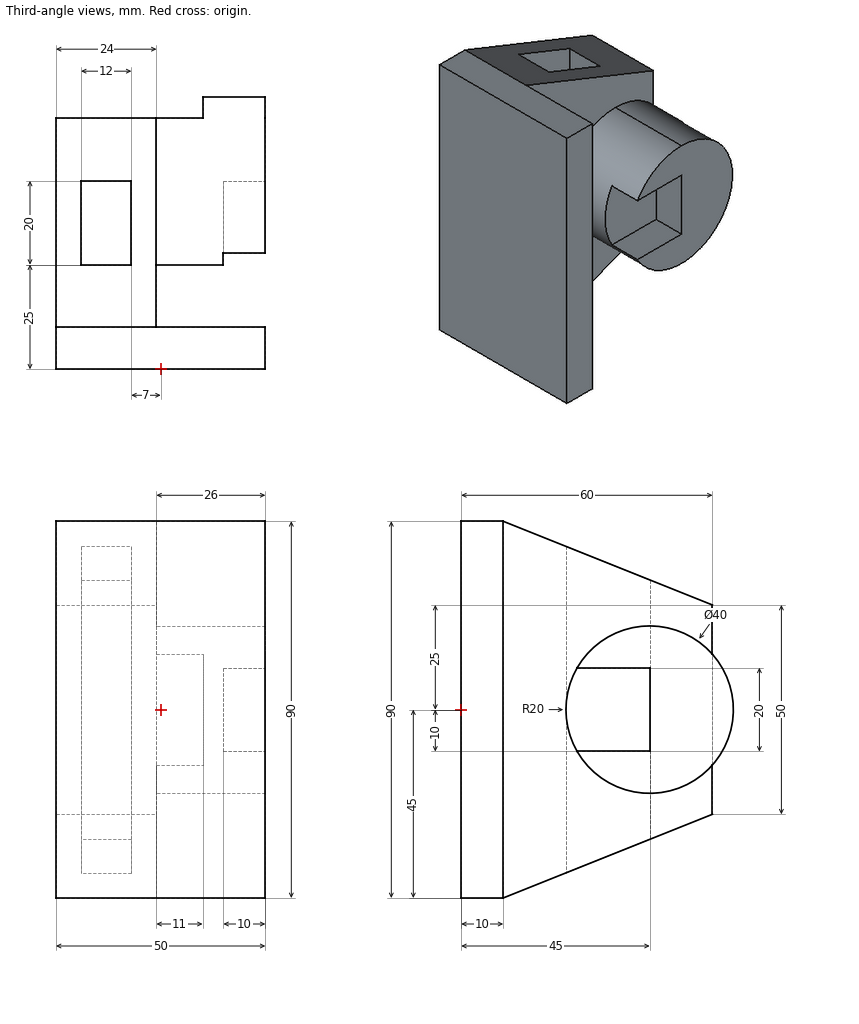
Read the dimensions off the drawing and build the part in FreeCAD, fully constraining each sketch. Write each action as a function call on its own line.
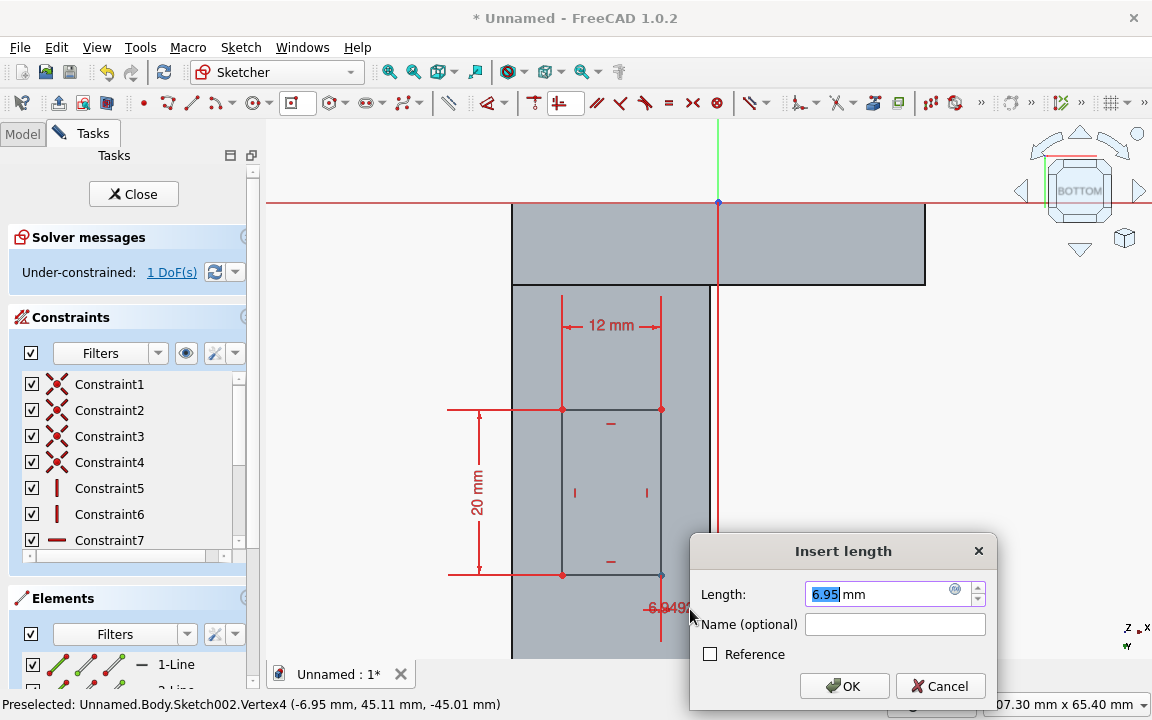
text(7)
key(Return)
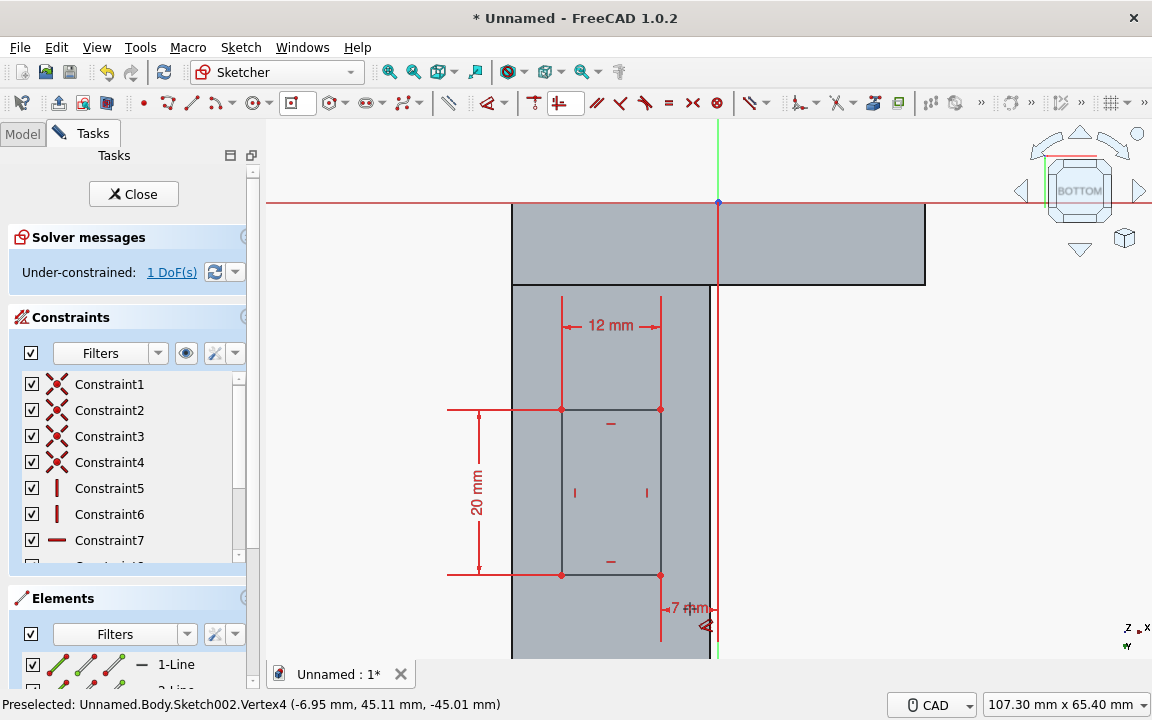
click(562, 410)
click(752, 306)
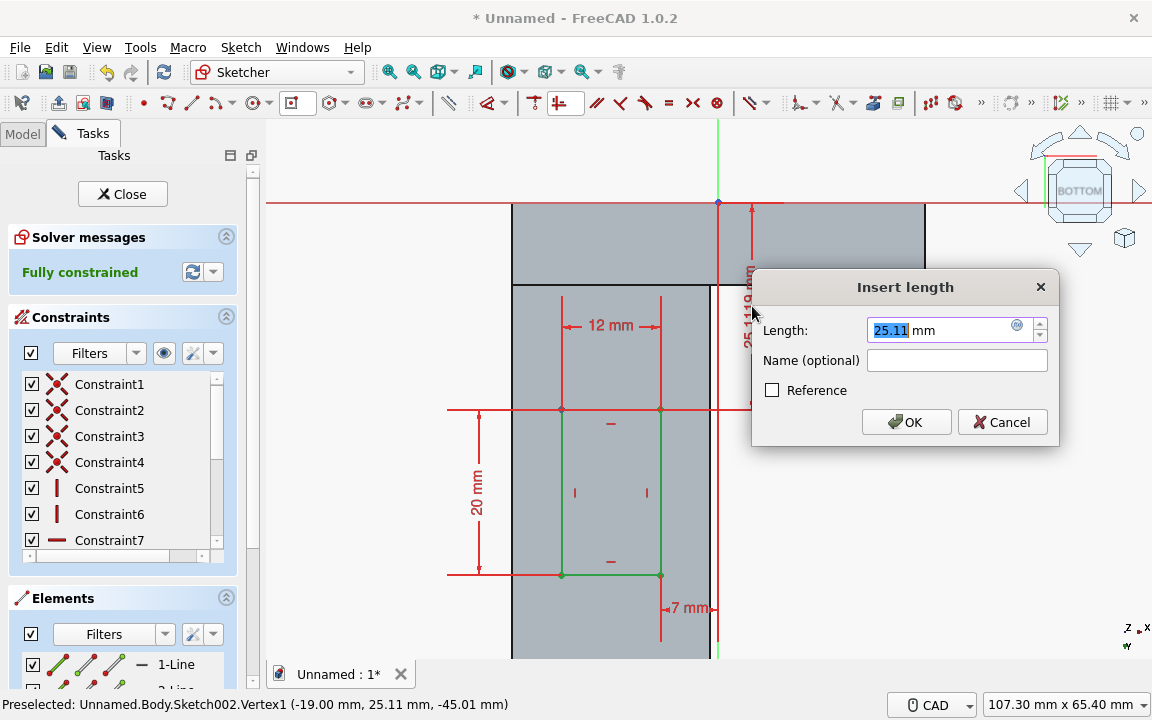
text(25)
key(Return)
key(Escape)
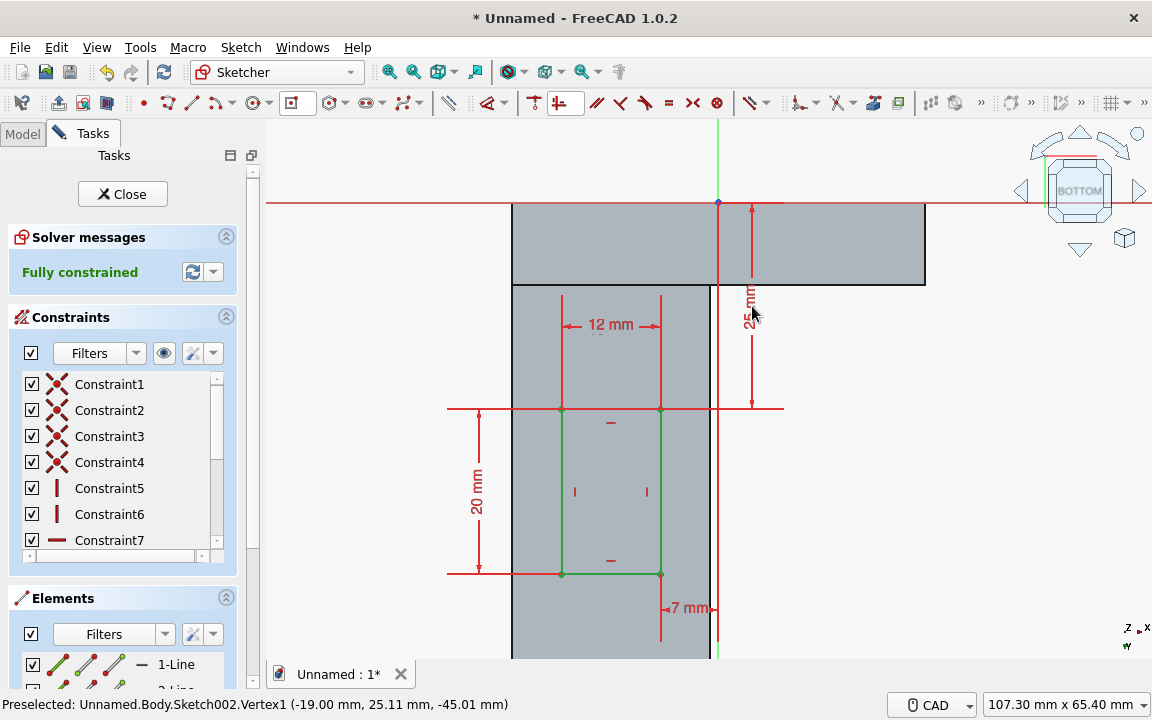
click(123, 194)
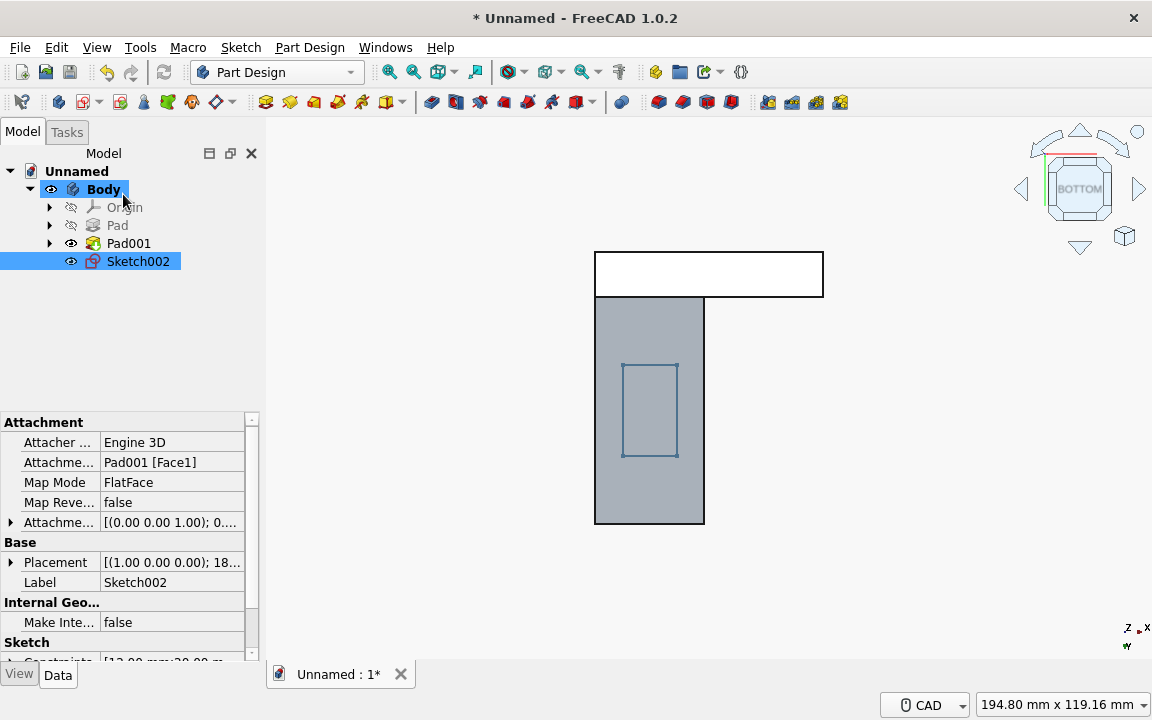
click(432, 102)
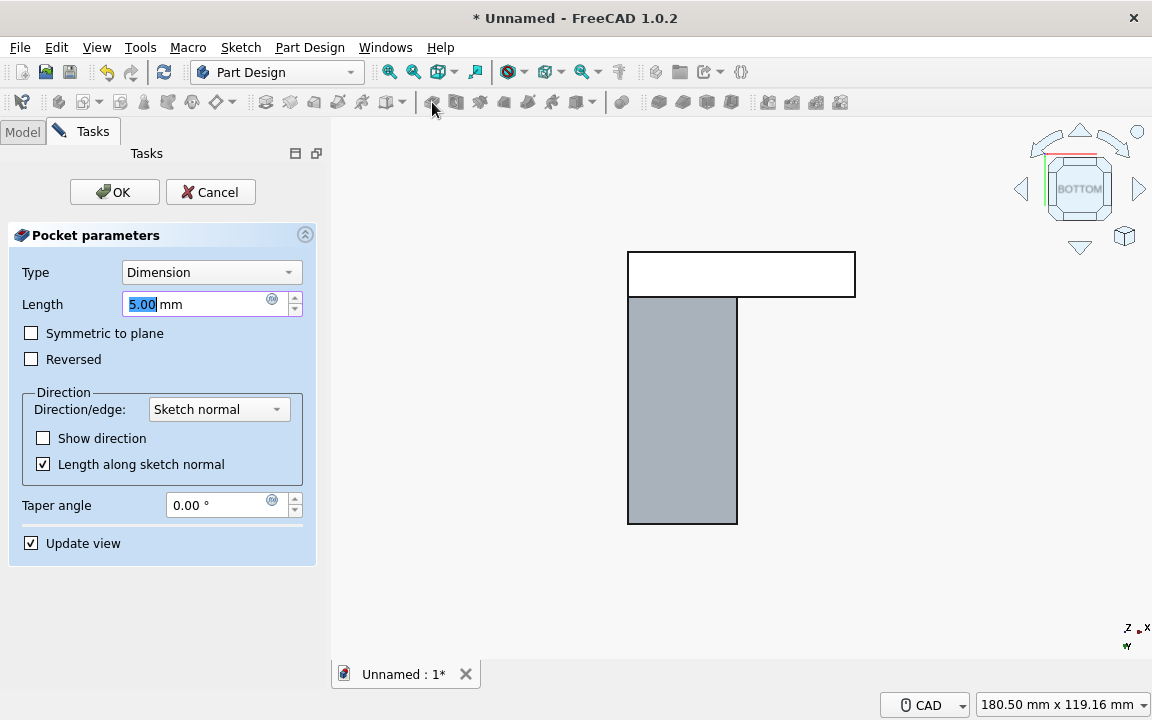
click(212, 272)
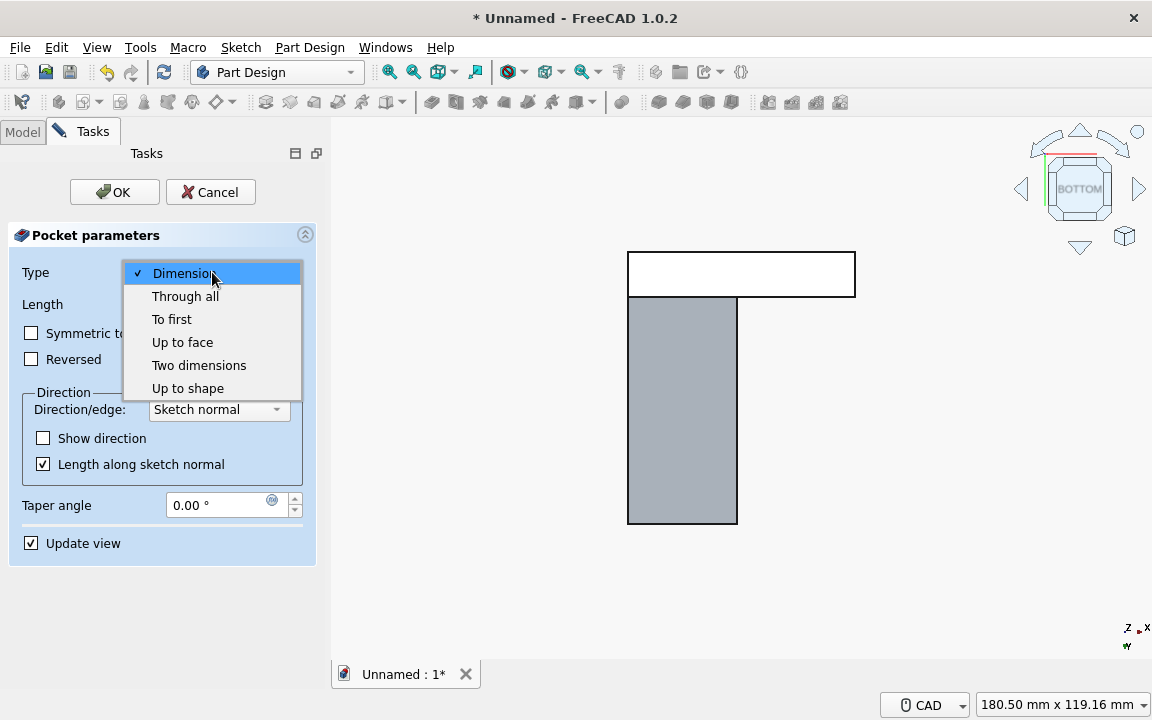
click(212, 366)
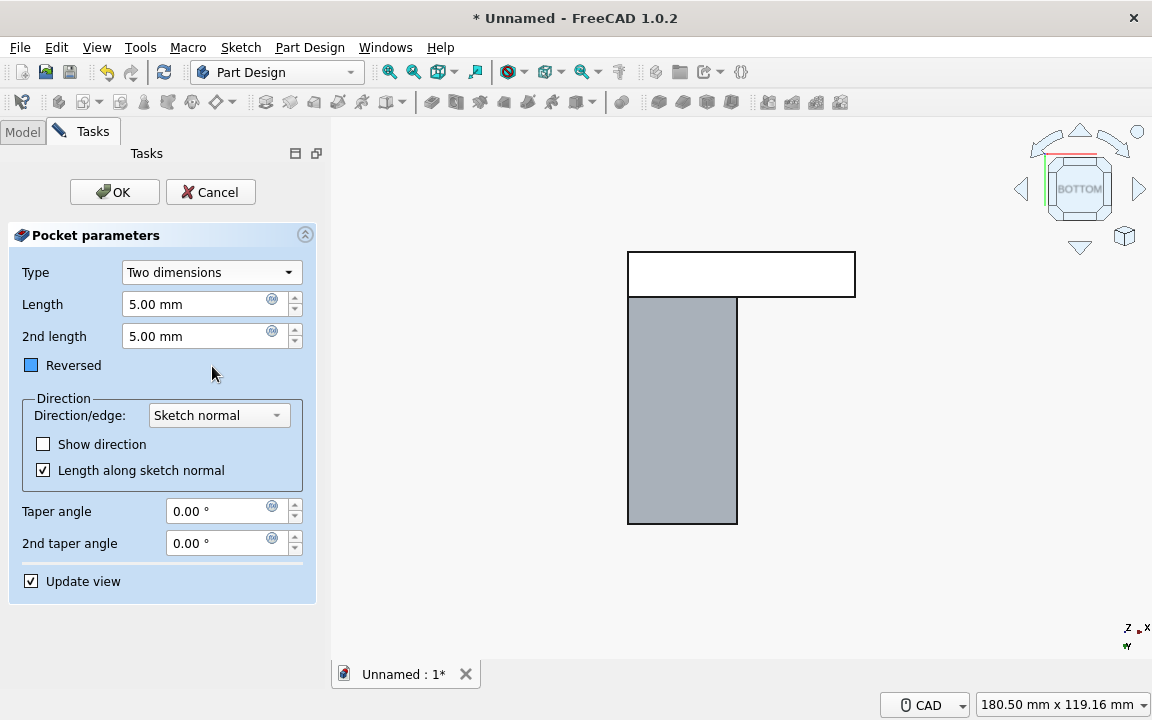
triple_click(204, 304)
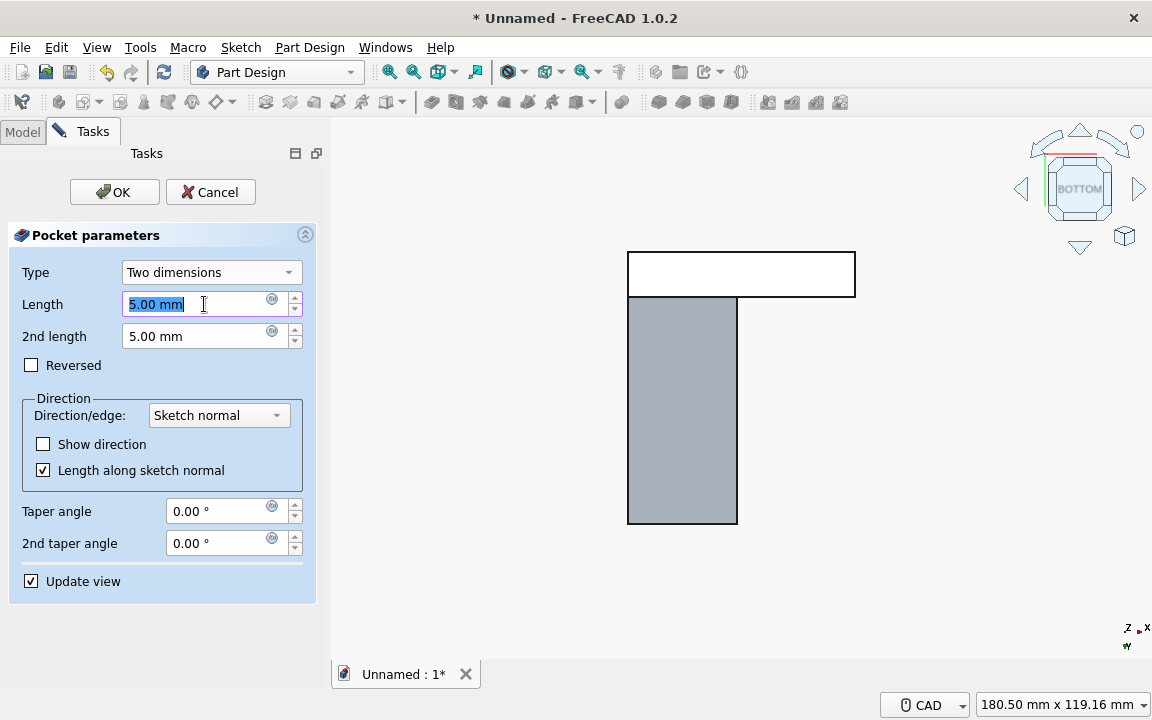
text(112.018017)
key(Tab)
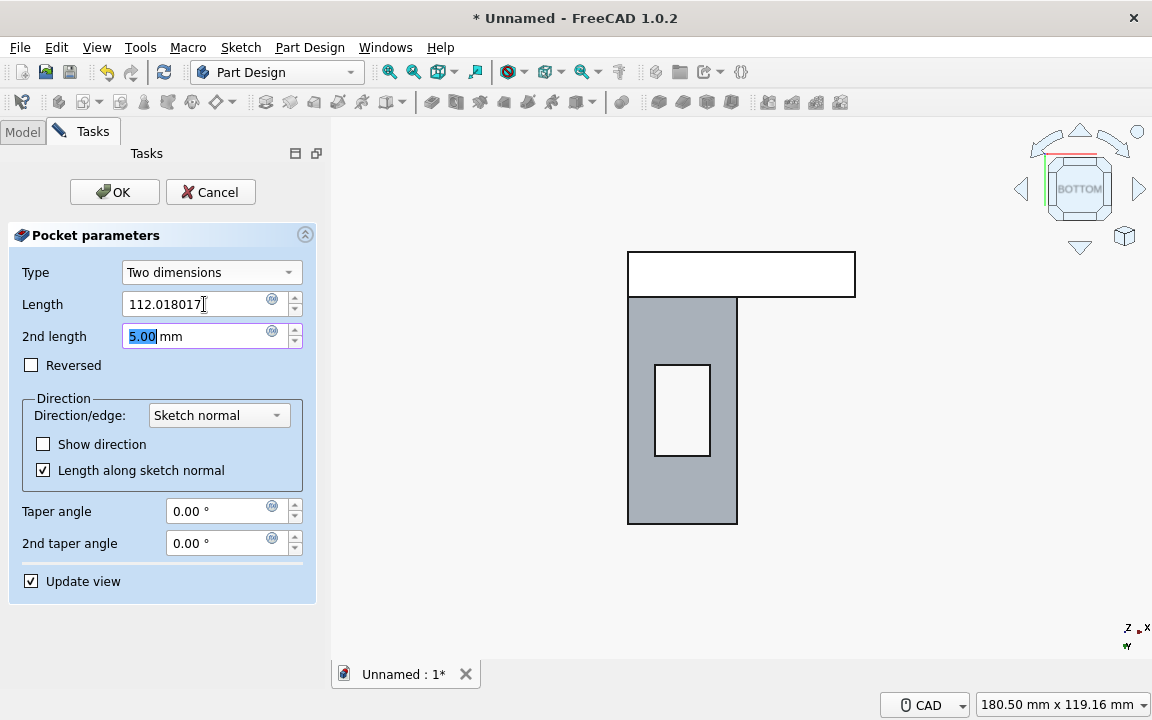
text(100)
key(Tab)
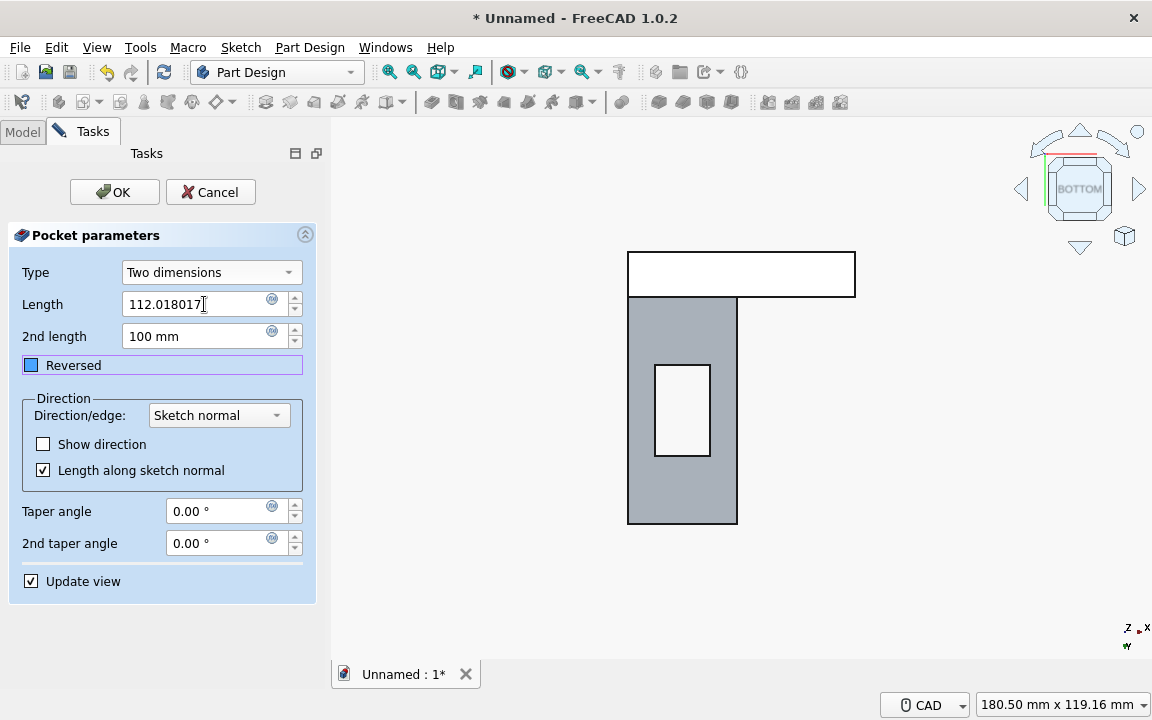
click(30, 365)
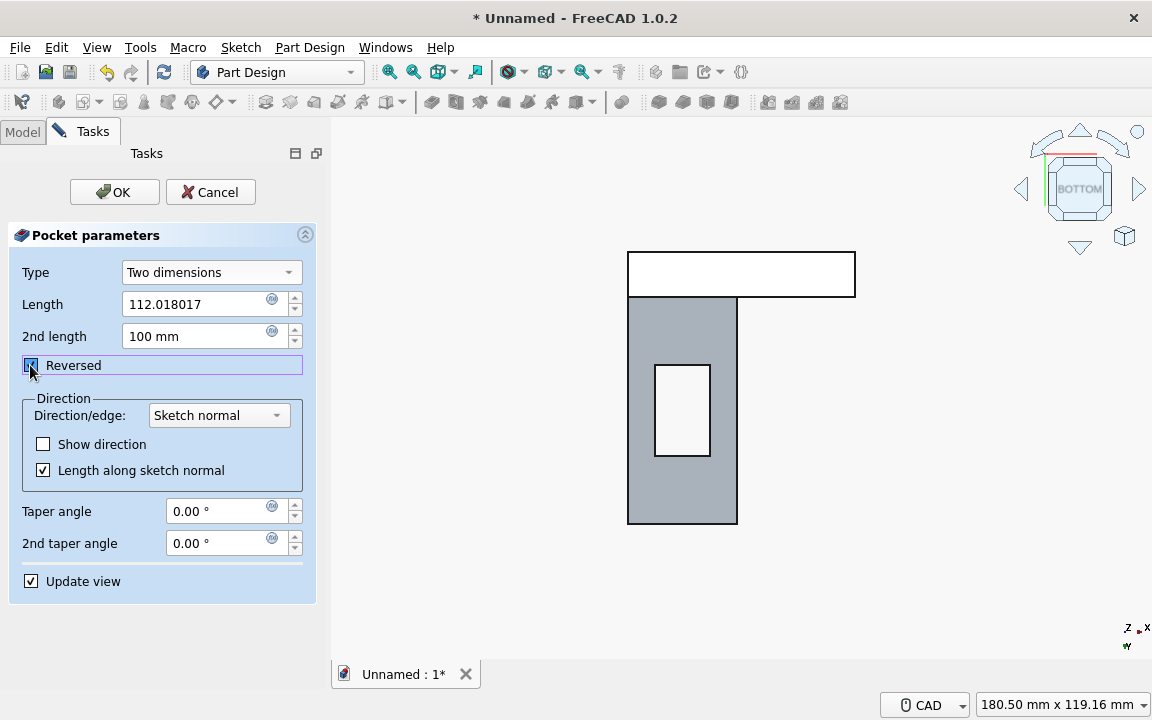
click(115, 192)